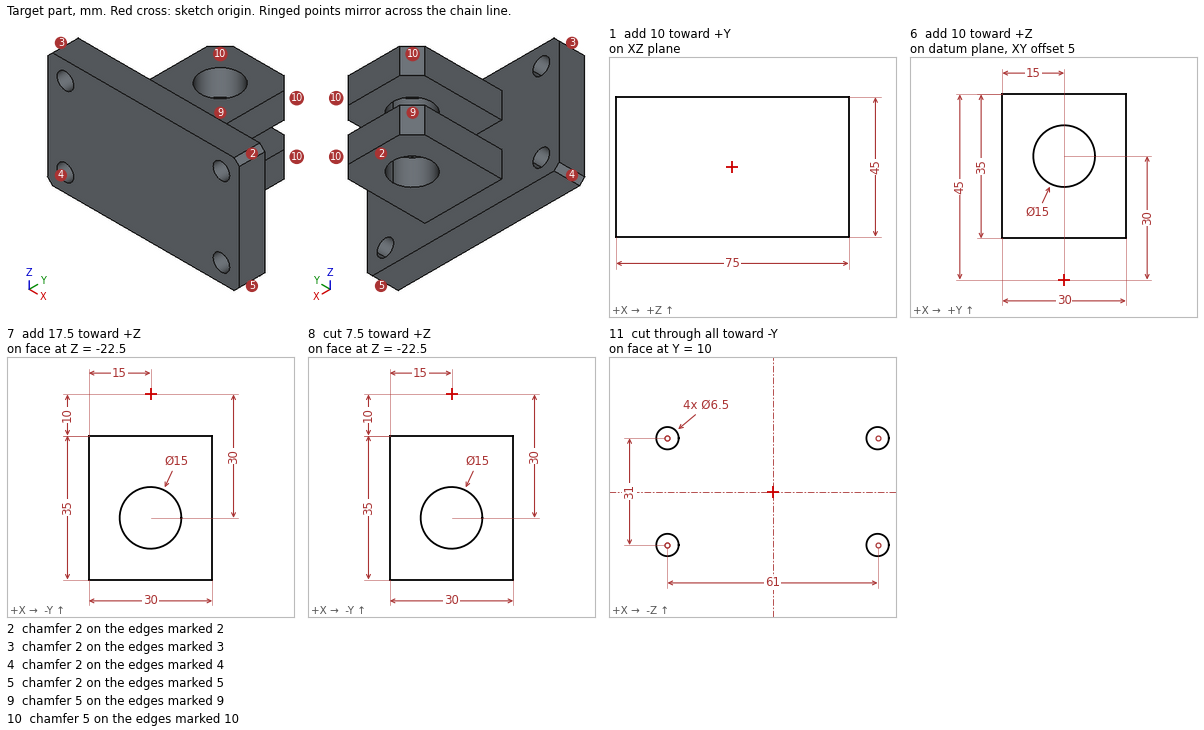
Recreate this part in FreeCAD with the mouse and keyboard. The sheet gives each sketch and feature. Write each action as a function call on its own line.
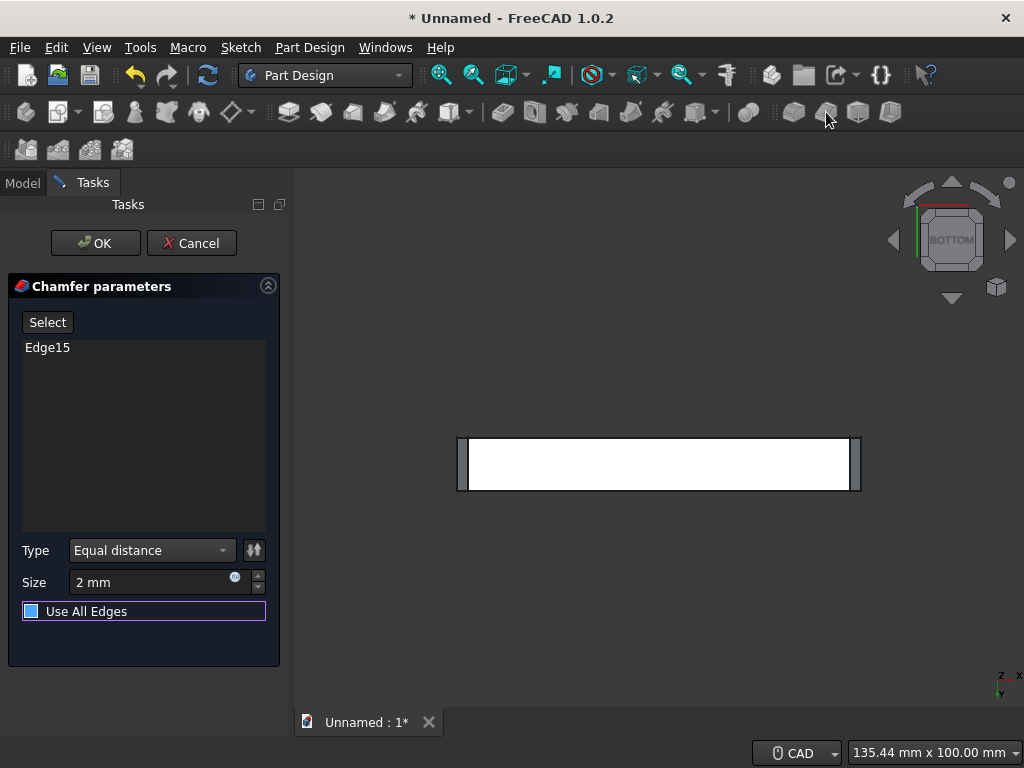
click(96, 243)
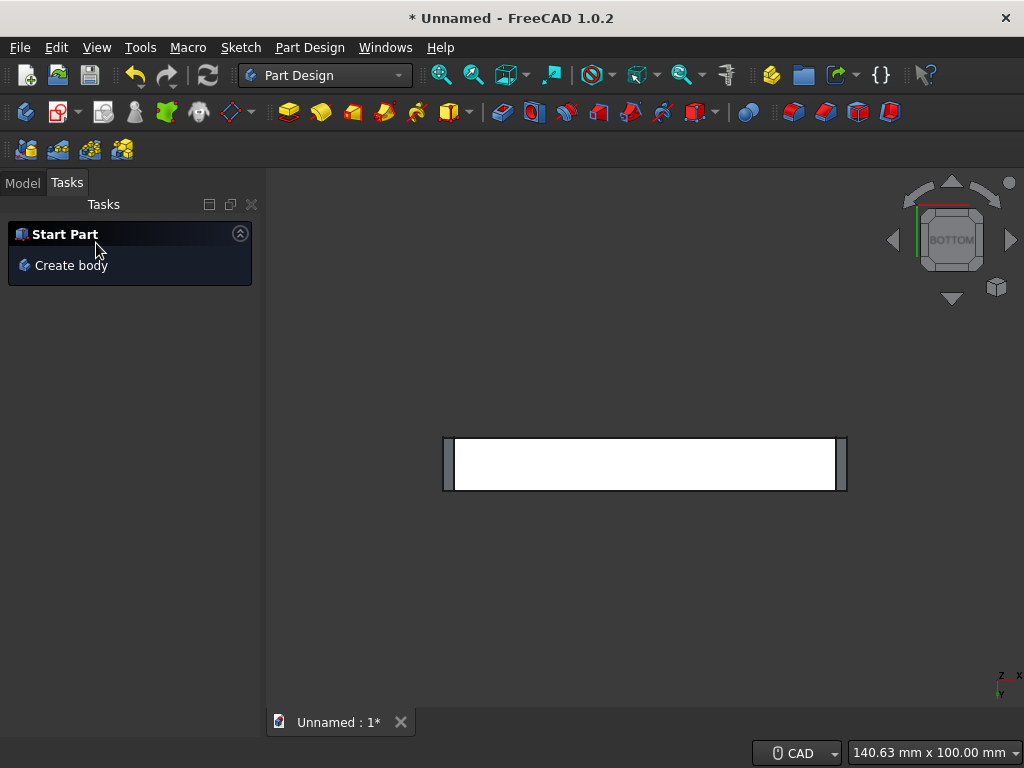
click(23, 182)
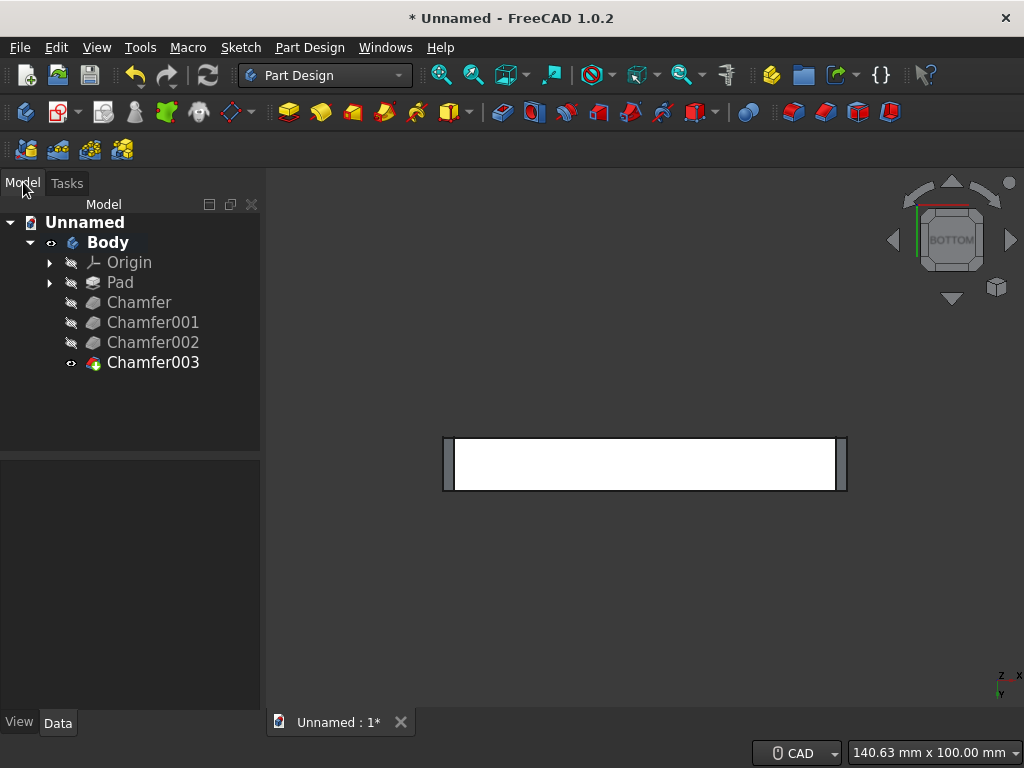
click(50, 263)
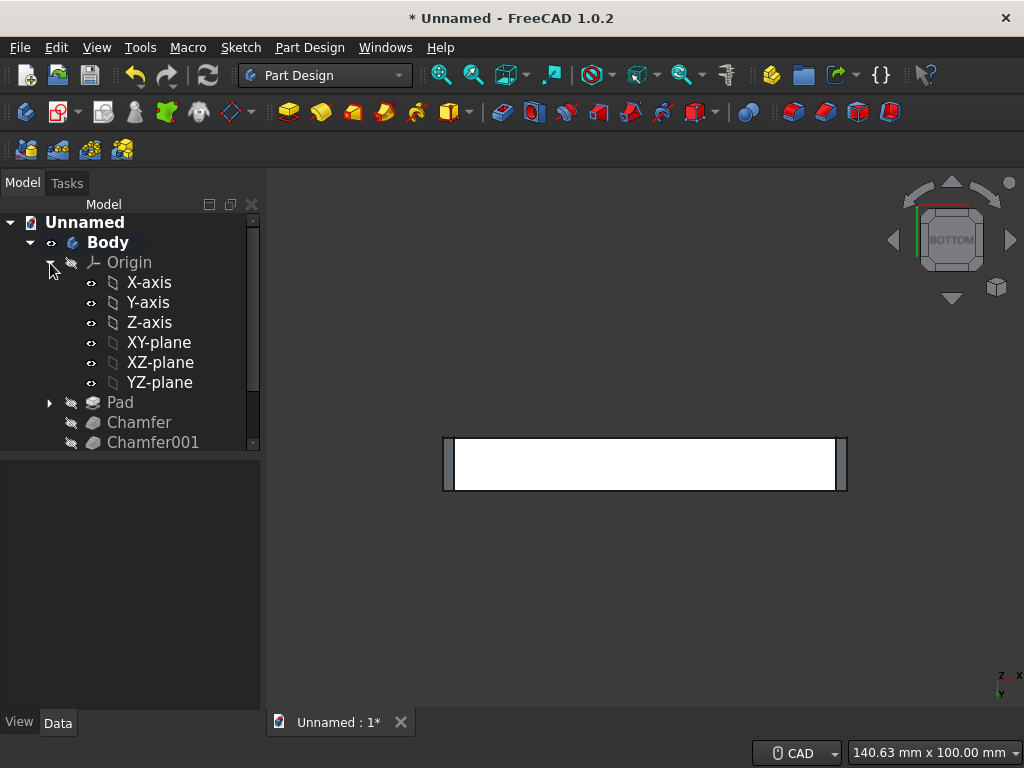
click(136, 343)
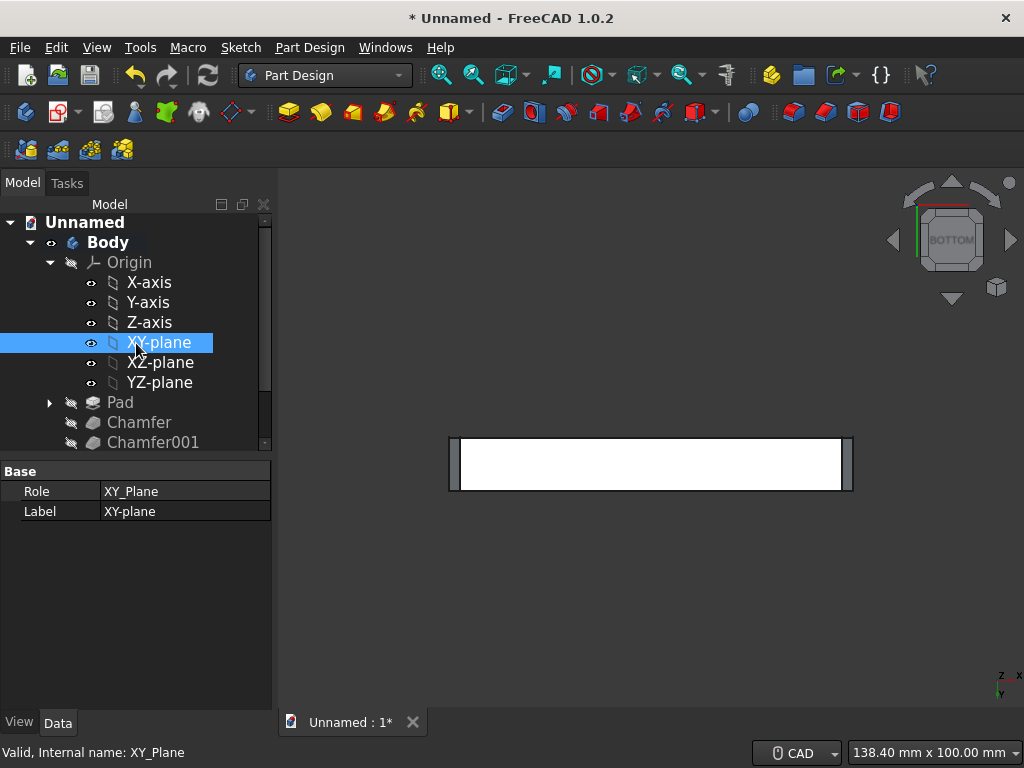
click(232, 112)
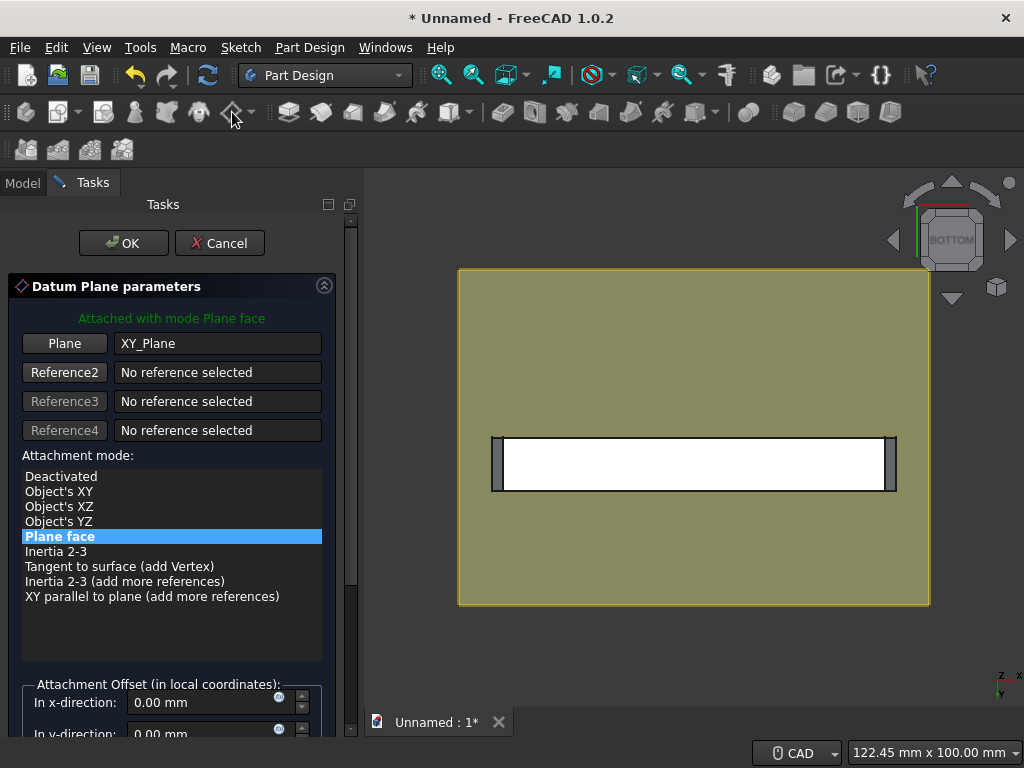
scroll(351, 475, down, 2)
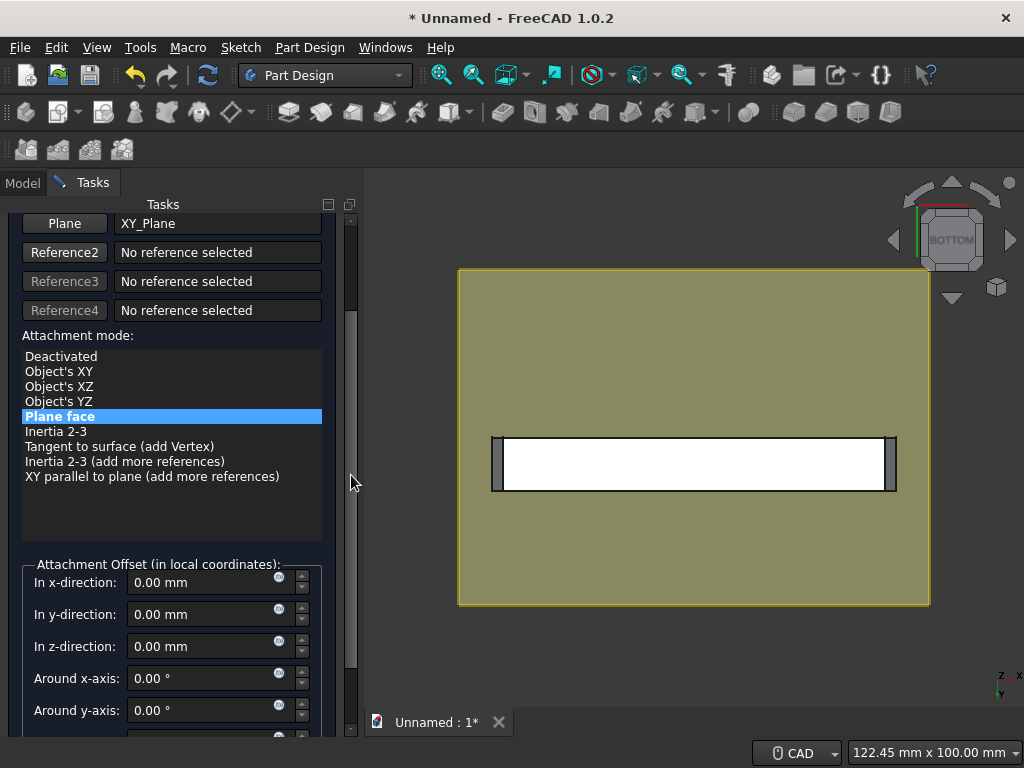
triple_click(210, 646)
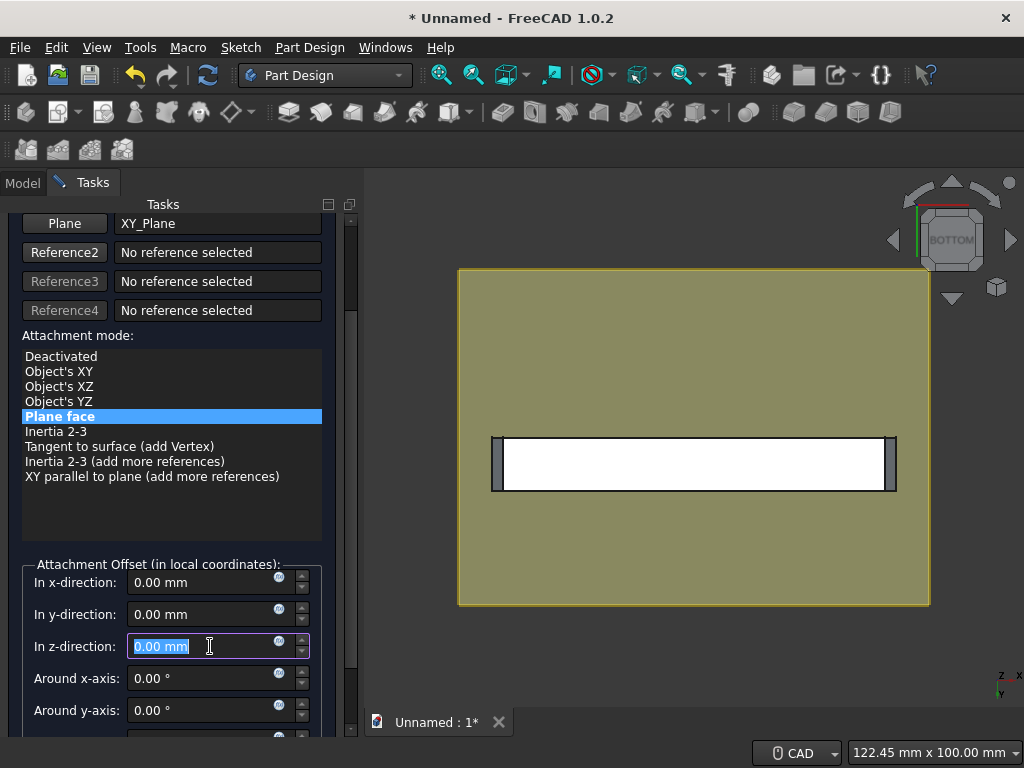
text(5)
key(Tab)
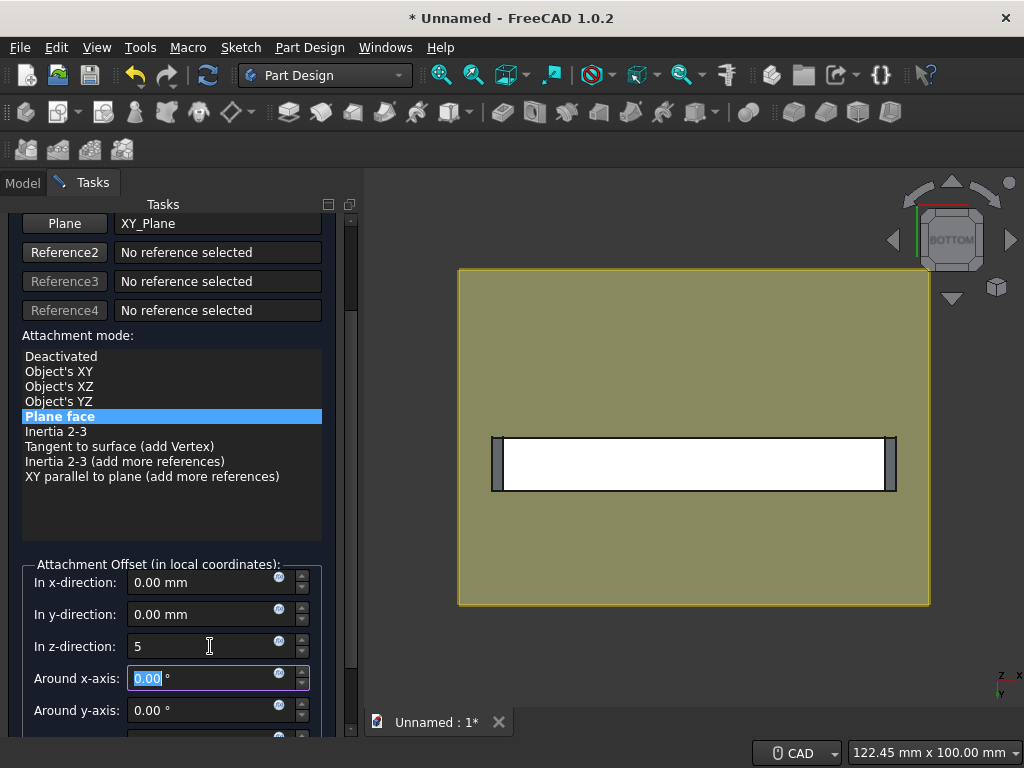
scroll(351, 475, up, 3)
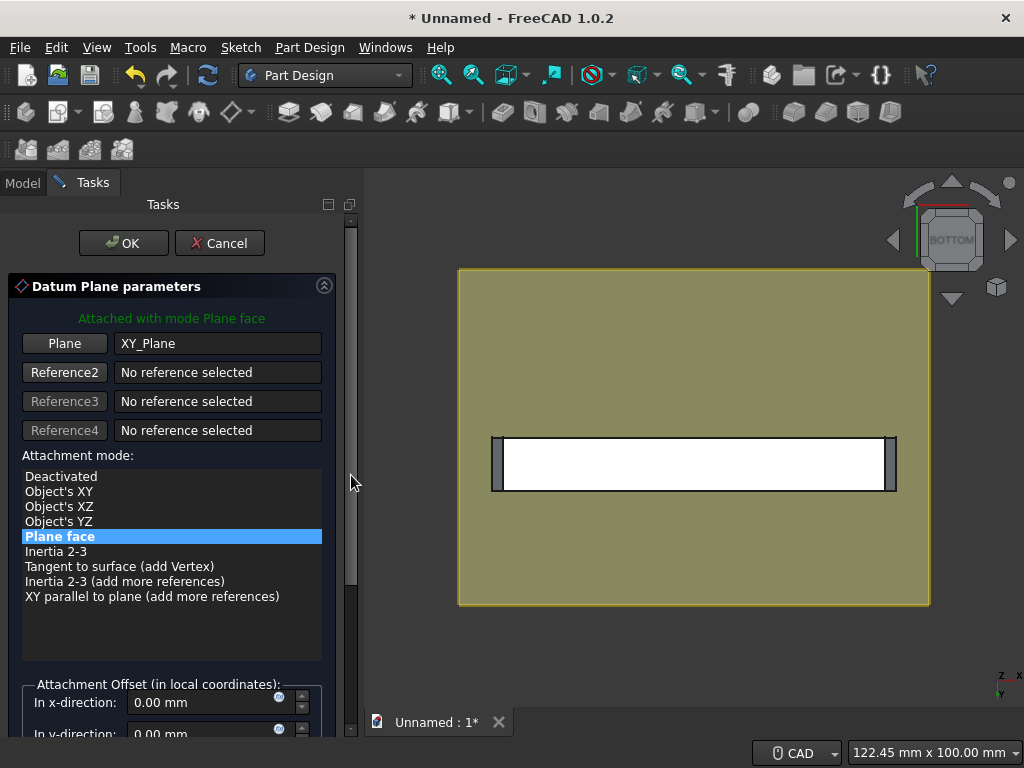
click(124, 243)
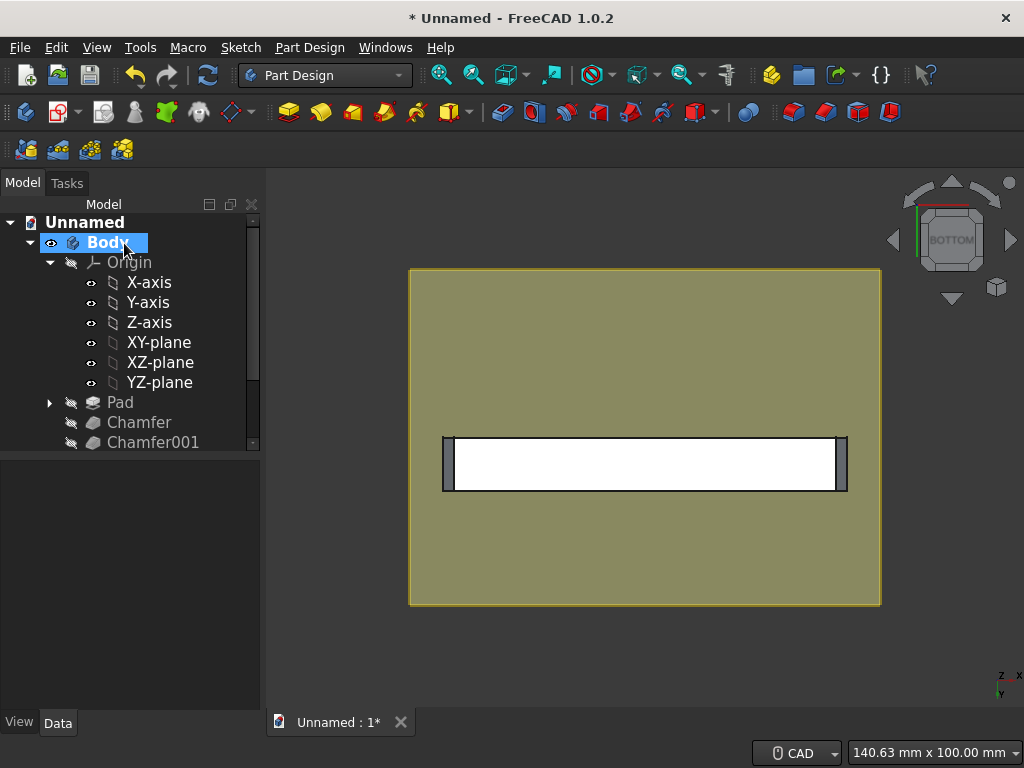
scroll(100, 338, down, 3)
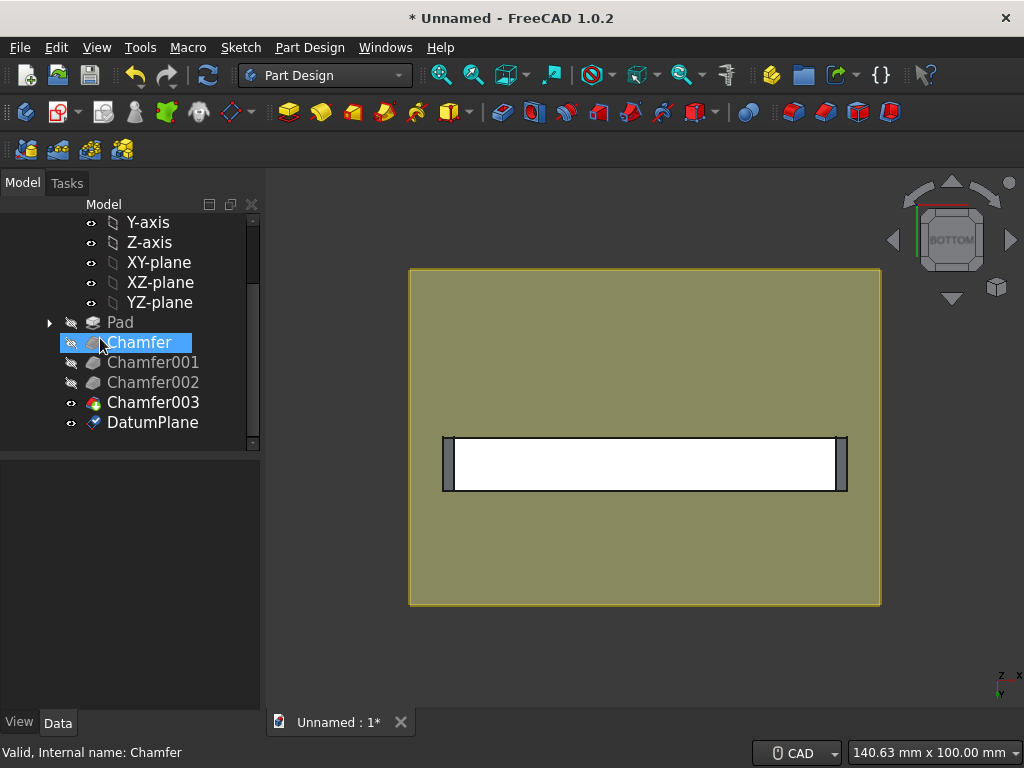
click(116, 423)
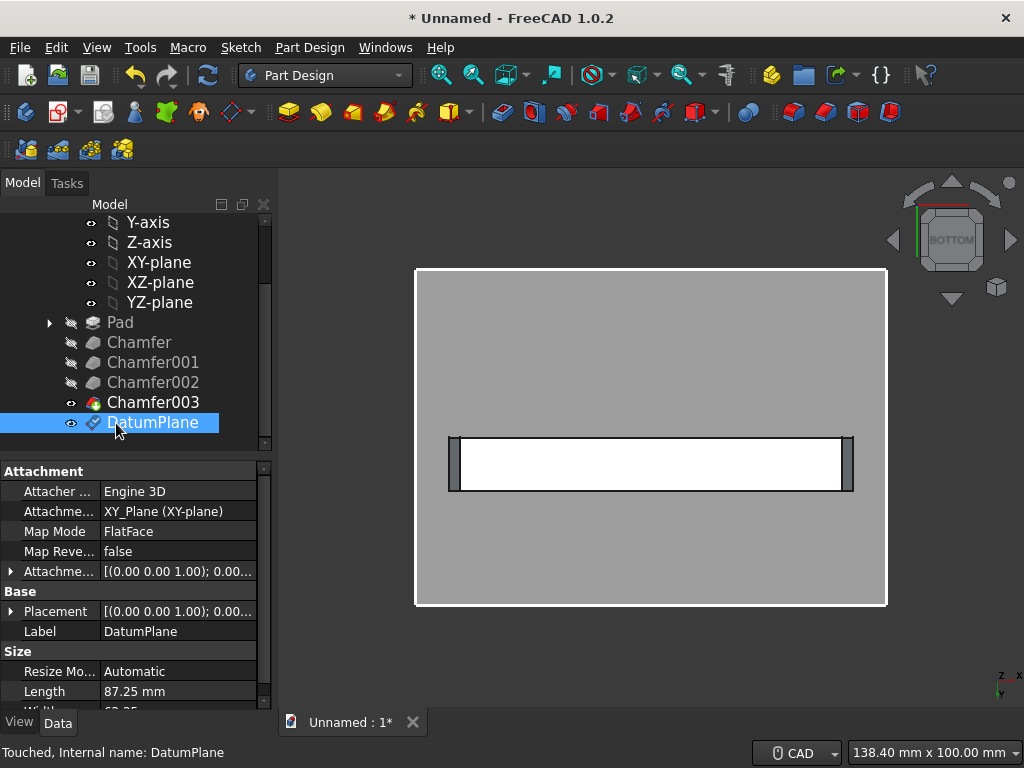
click(58, 112)